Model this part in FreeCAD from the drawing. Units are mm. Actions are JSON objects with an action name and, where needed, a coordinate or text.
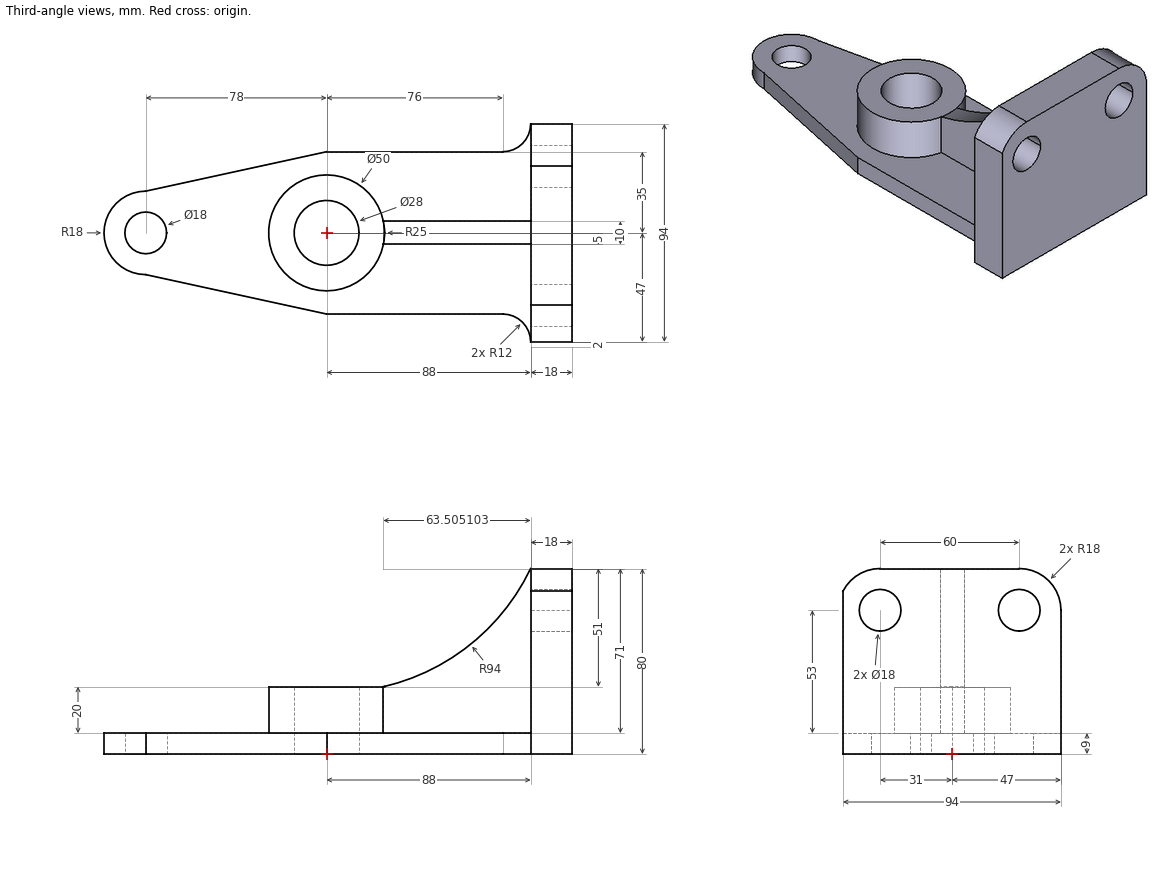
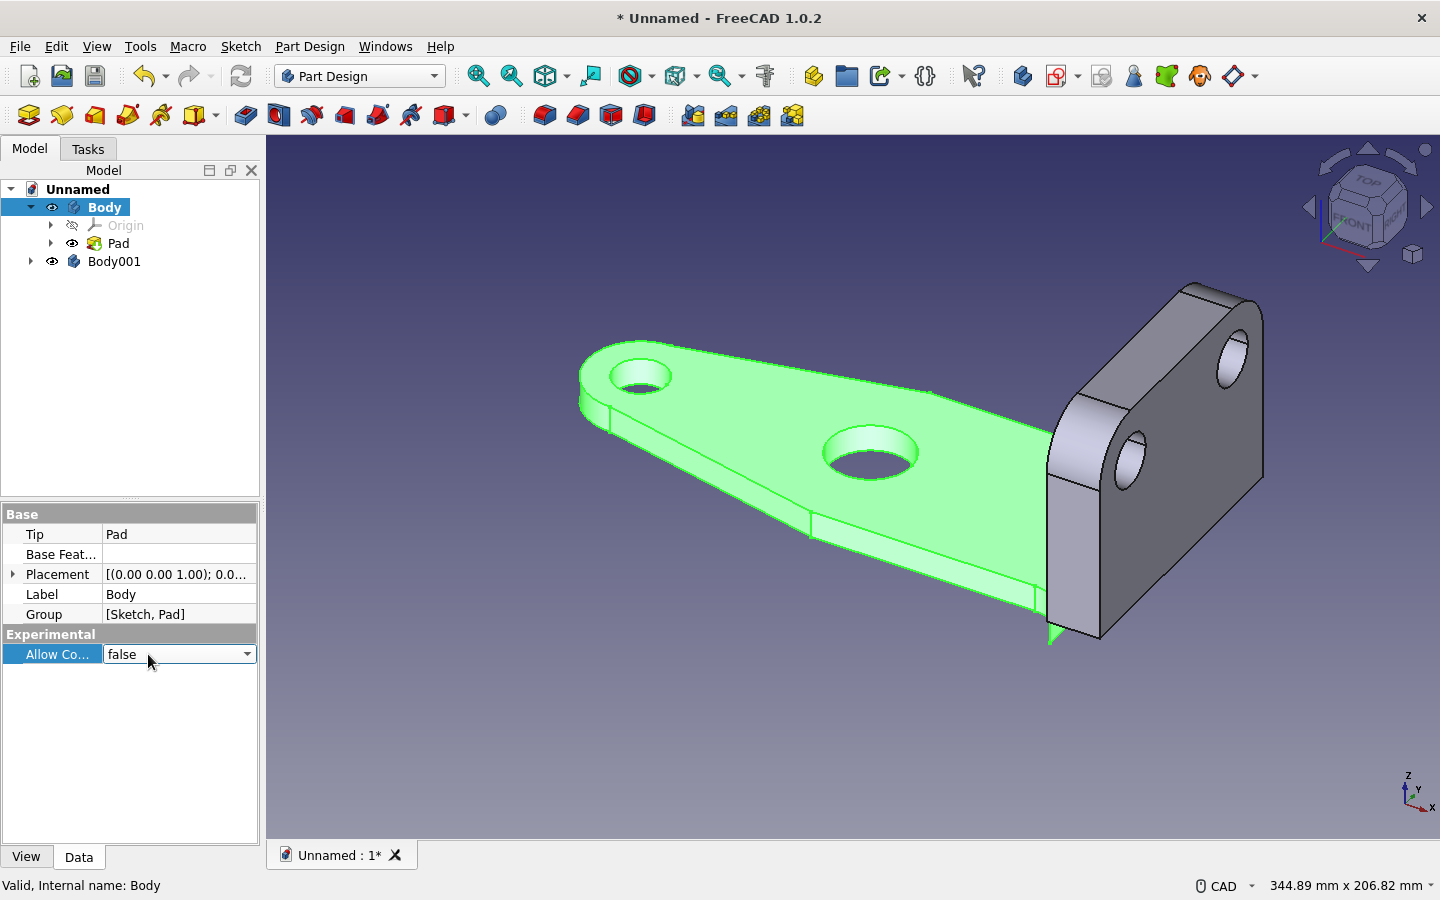
{"action": "left_click", "coordinate": [148, 654]}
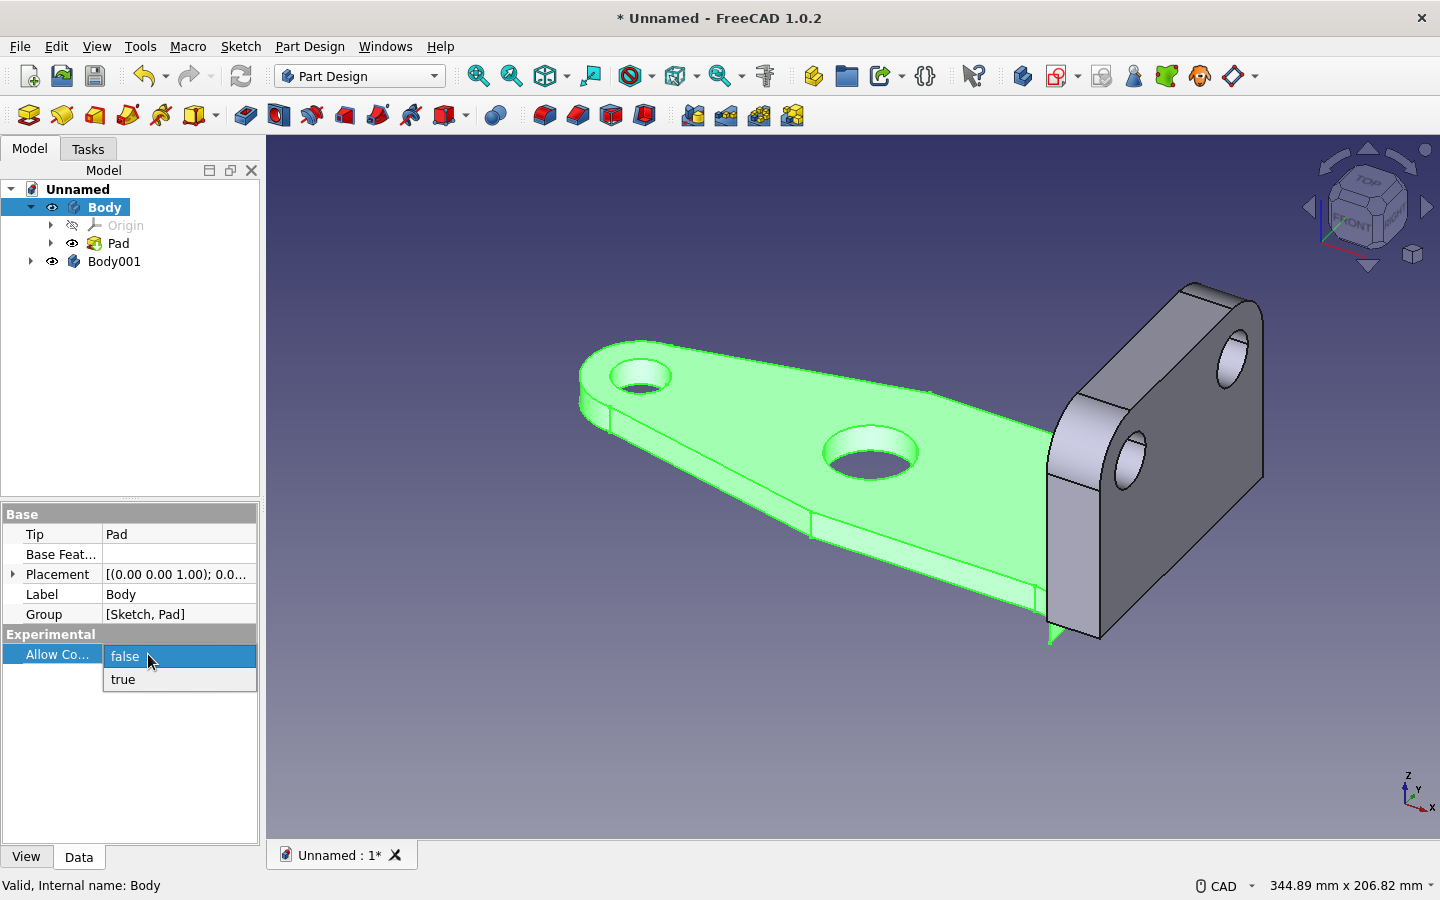
{"action": "left_click", "coordinate": [178, 680]}
{"action": "key", "text": "Return"}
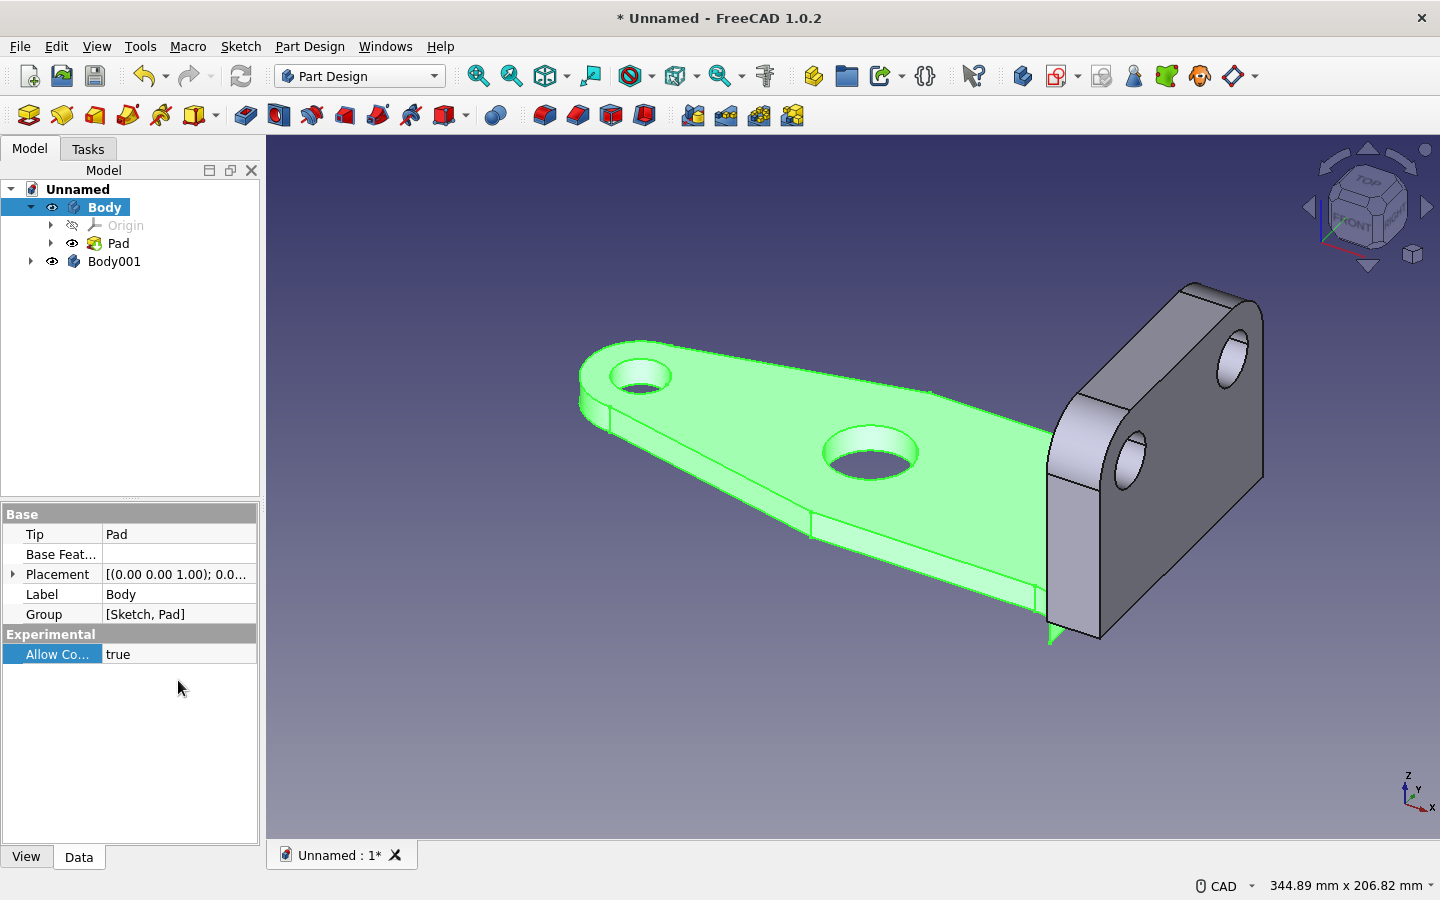
{"action": "left_click", "coordinate": [97, 261]}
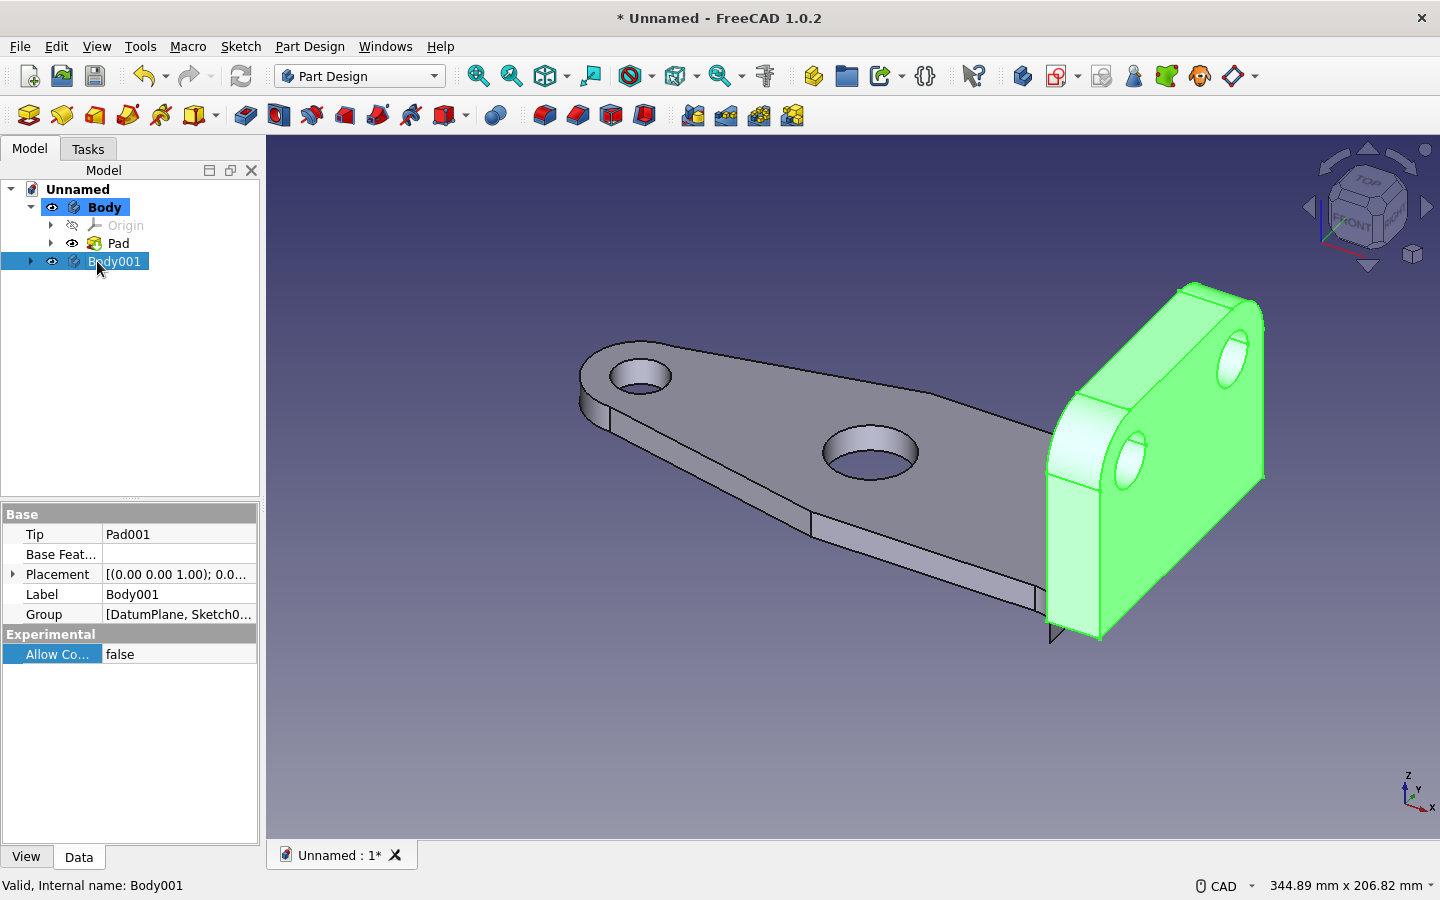
{"action": "left_click", "coordinate": [496, 116]}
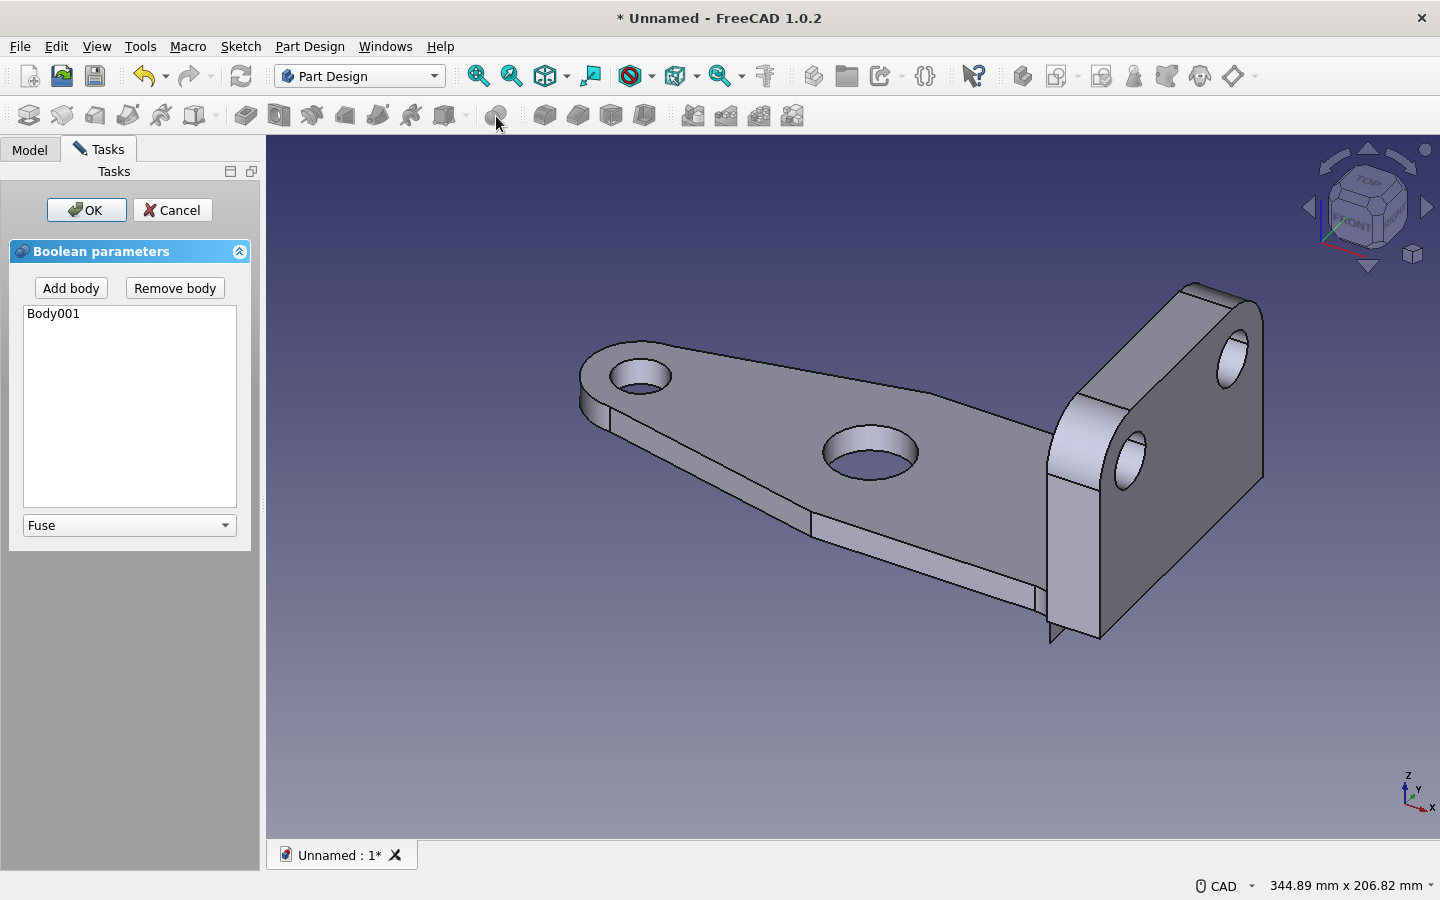
{"action": "left_click", "coordinate": [87, 210]}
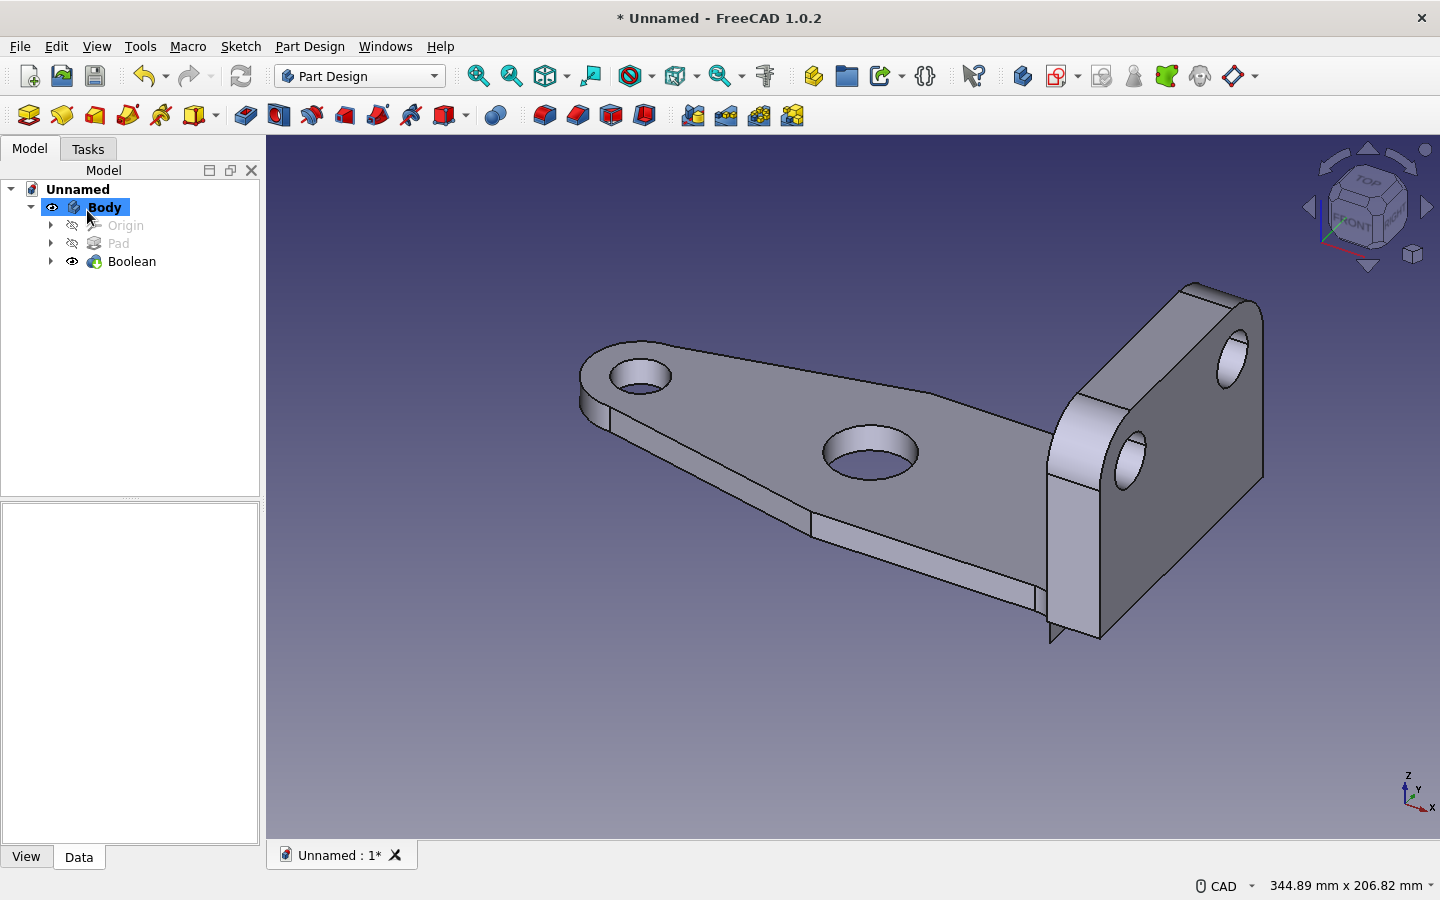
{"action": "left_click", "coordinate": [479, 76]}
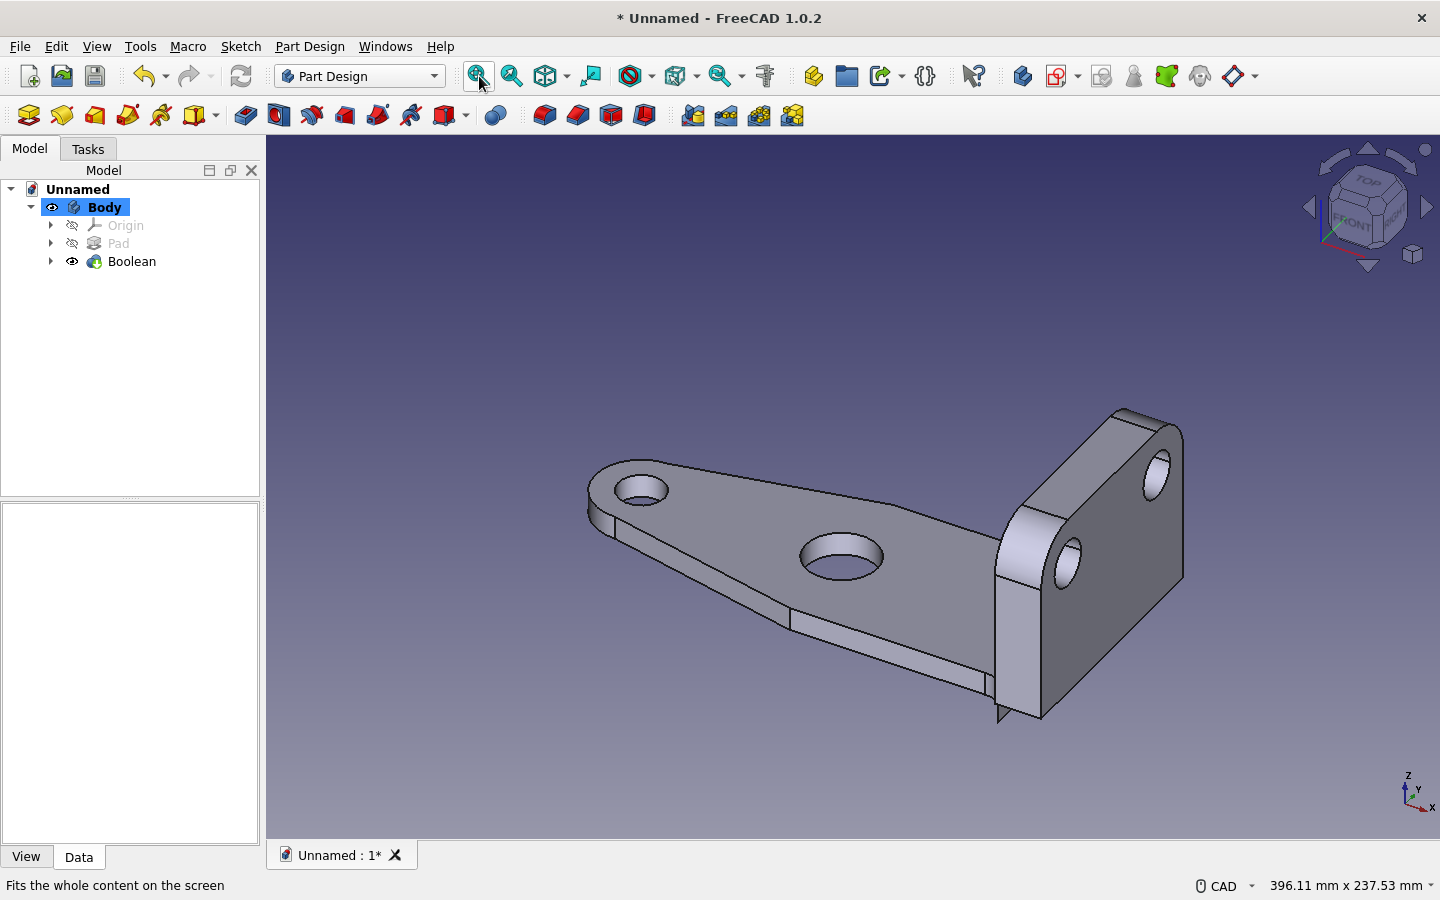
{"action": "key", "text": "6"}